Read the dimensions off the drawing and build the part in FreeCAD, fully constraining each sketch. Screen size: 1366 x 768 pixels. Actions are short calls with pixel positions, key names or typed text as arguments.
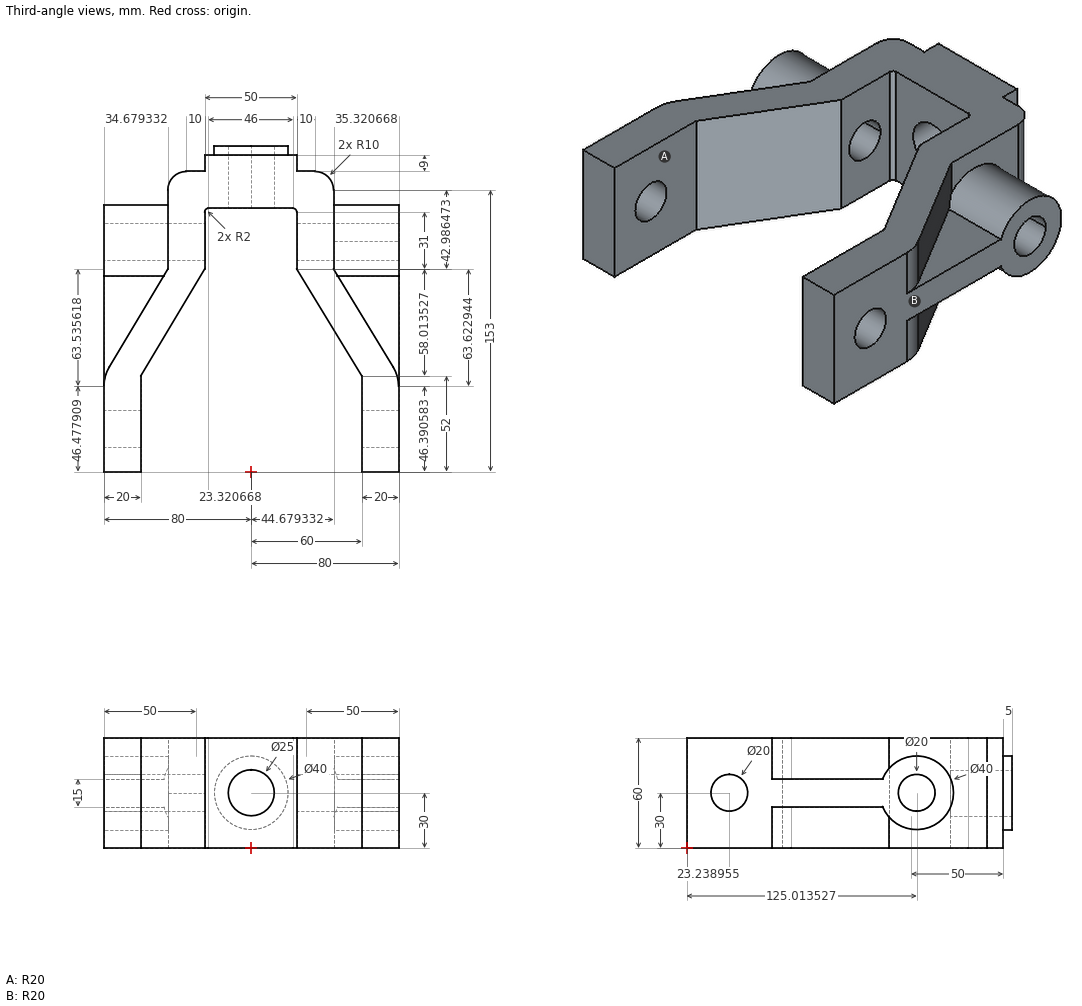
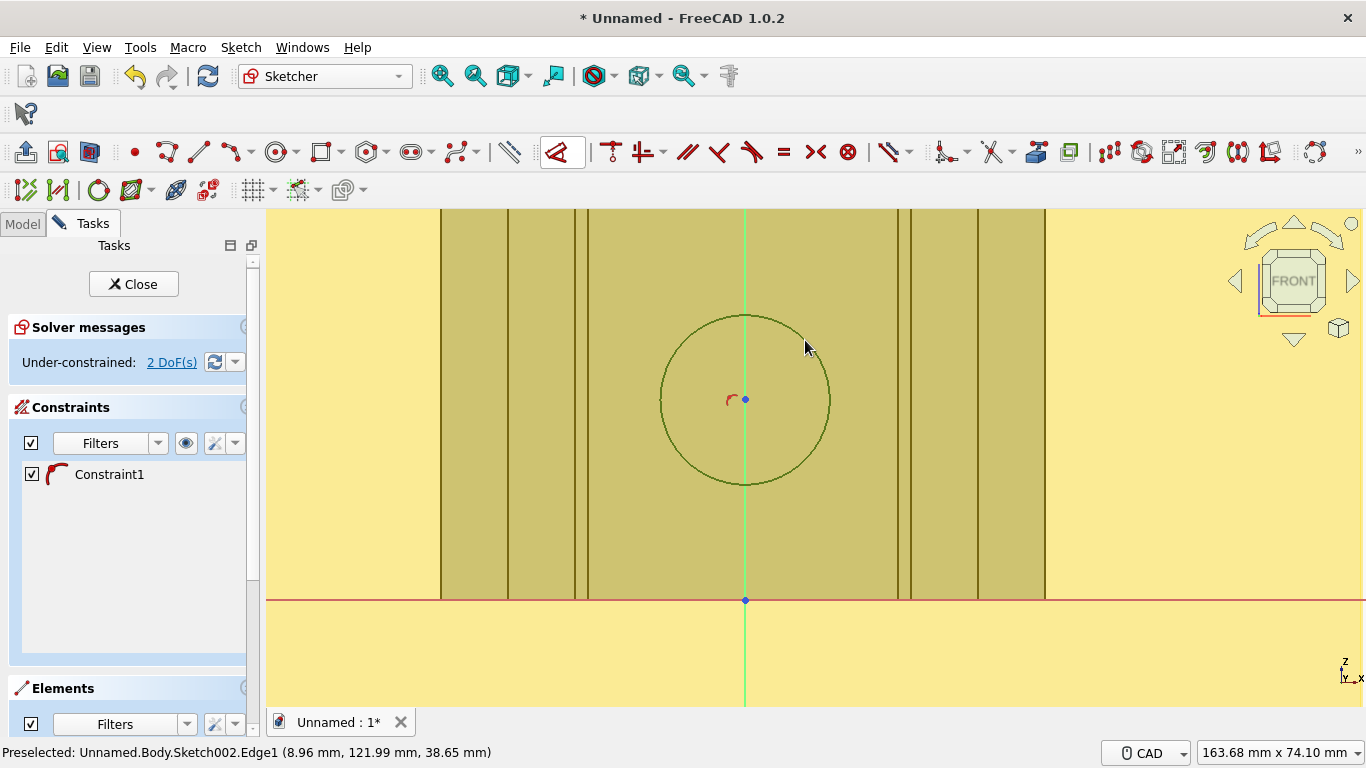
key(k)
key(o)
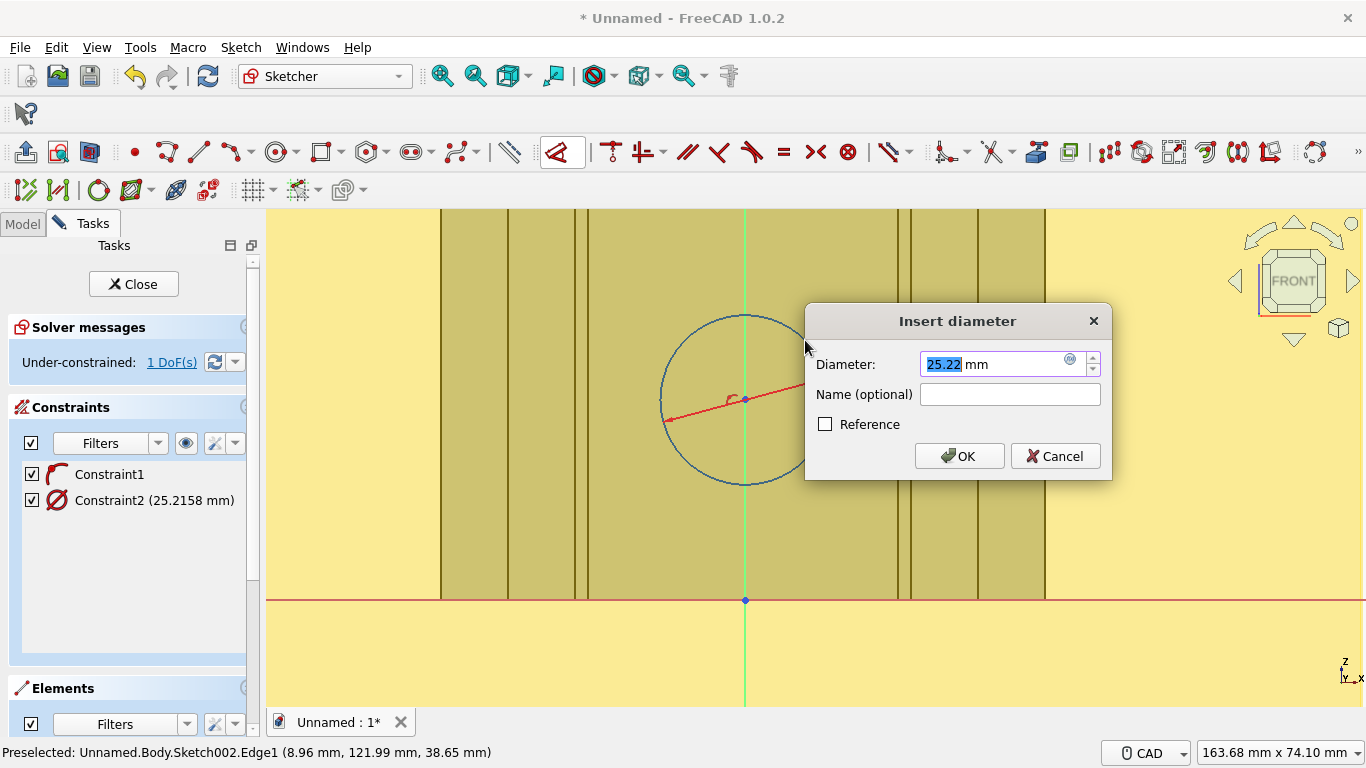
text(25)
key(Return)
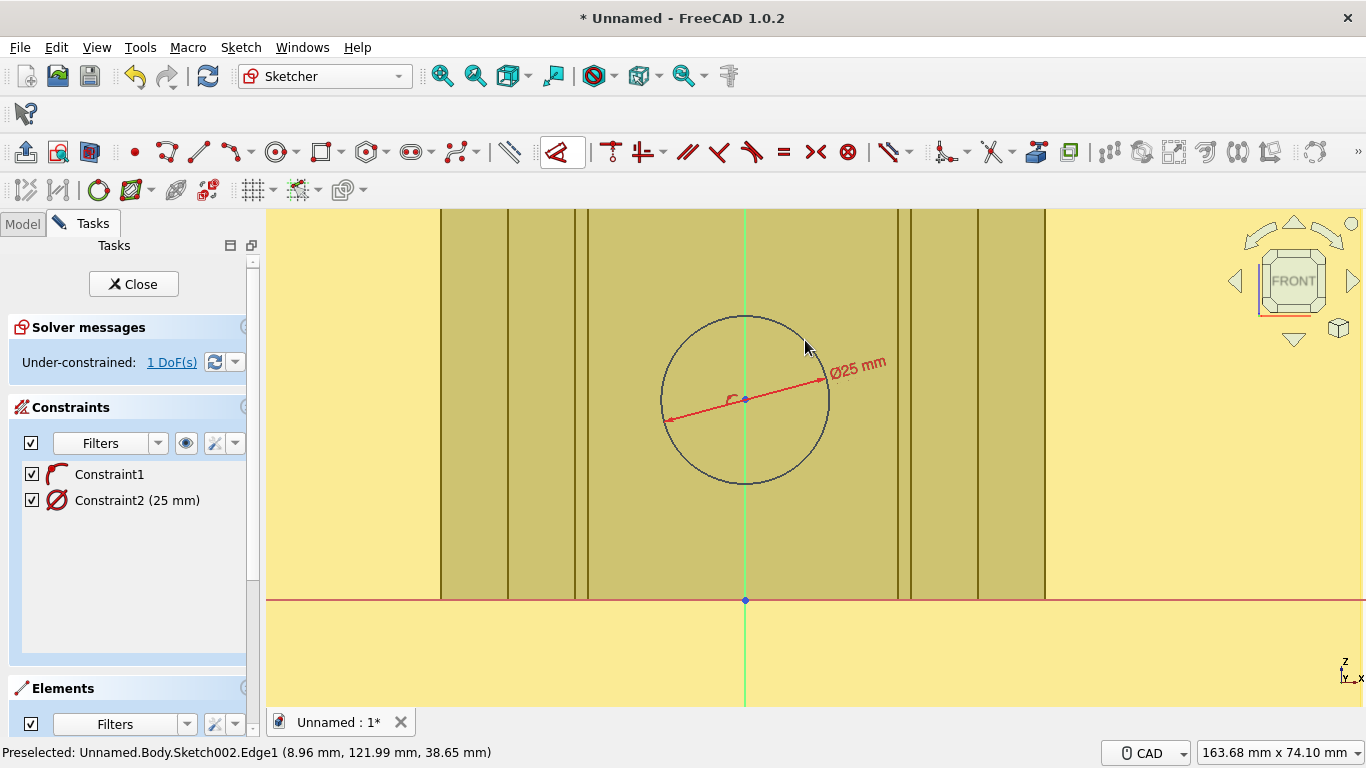
click(745, 400)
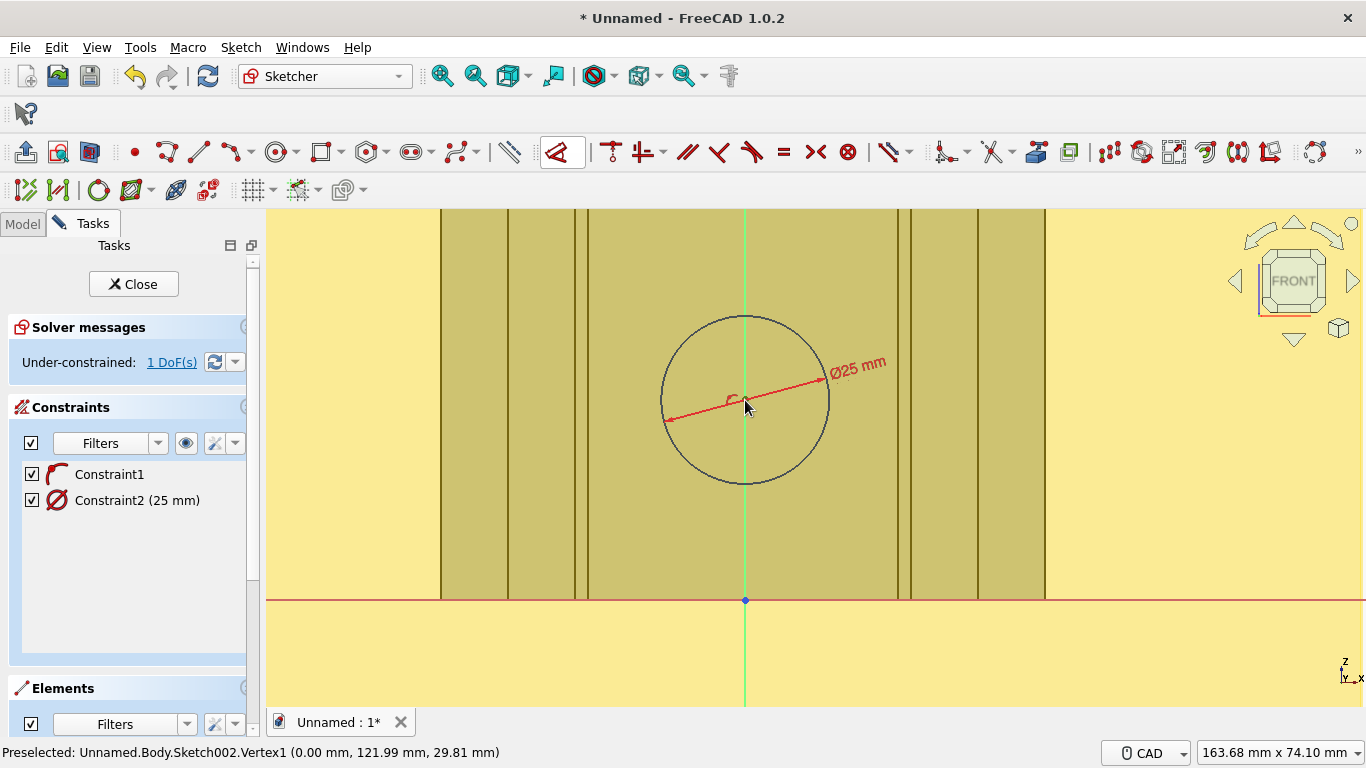
key(i)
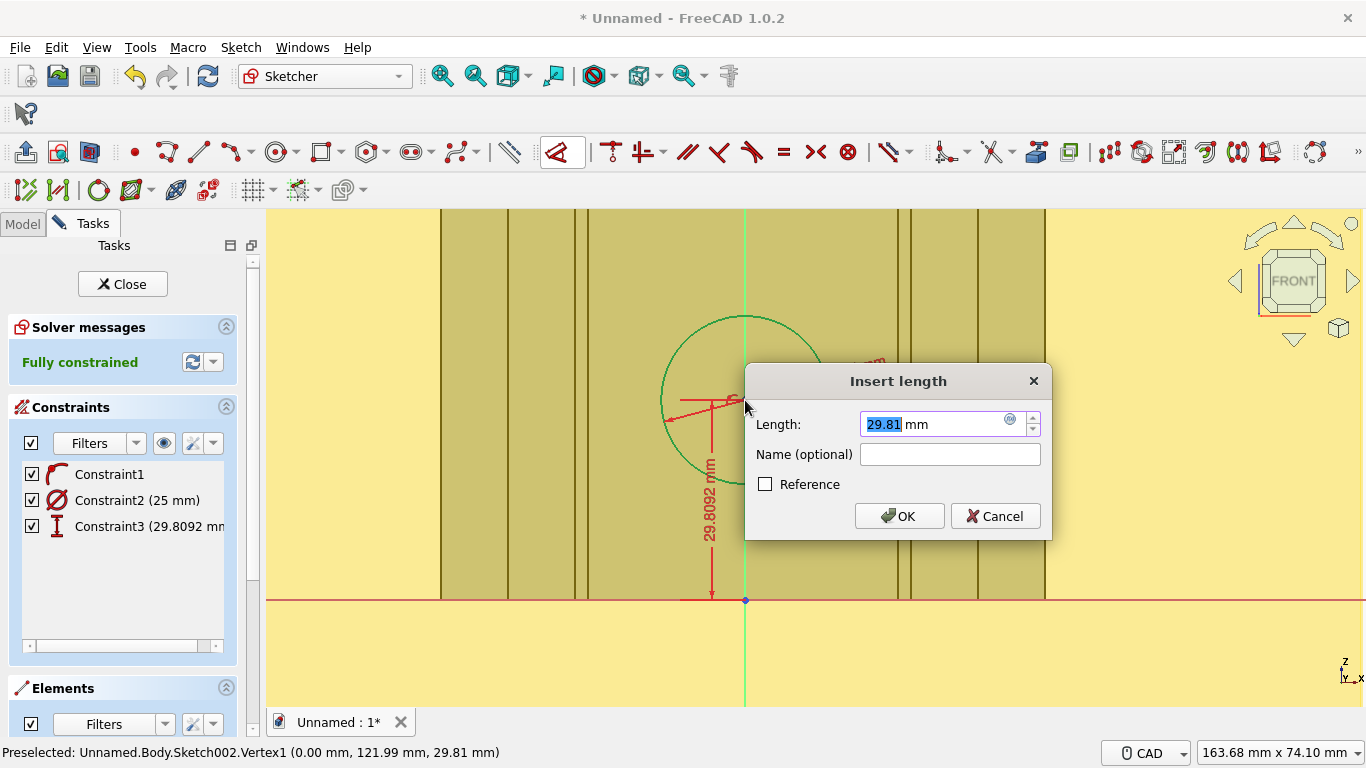
text(30)
key(Return)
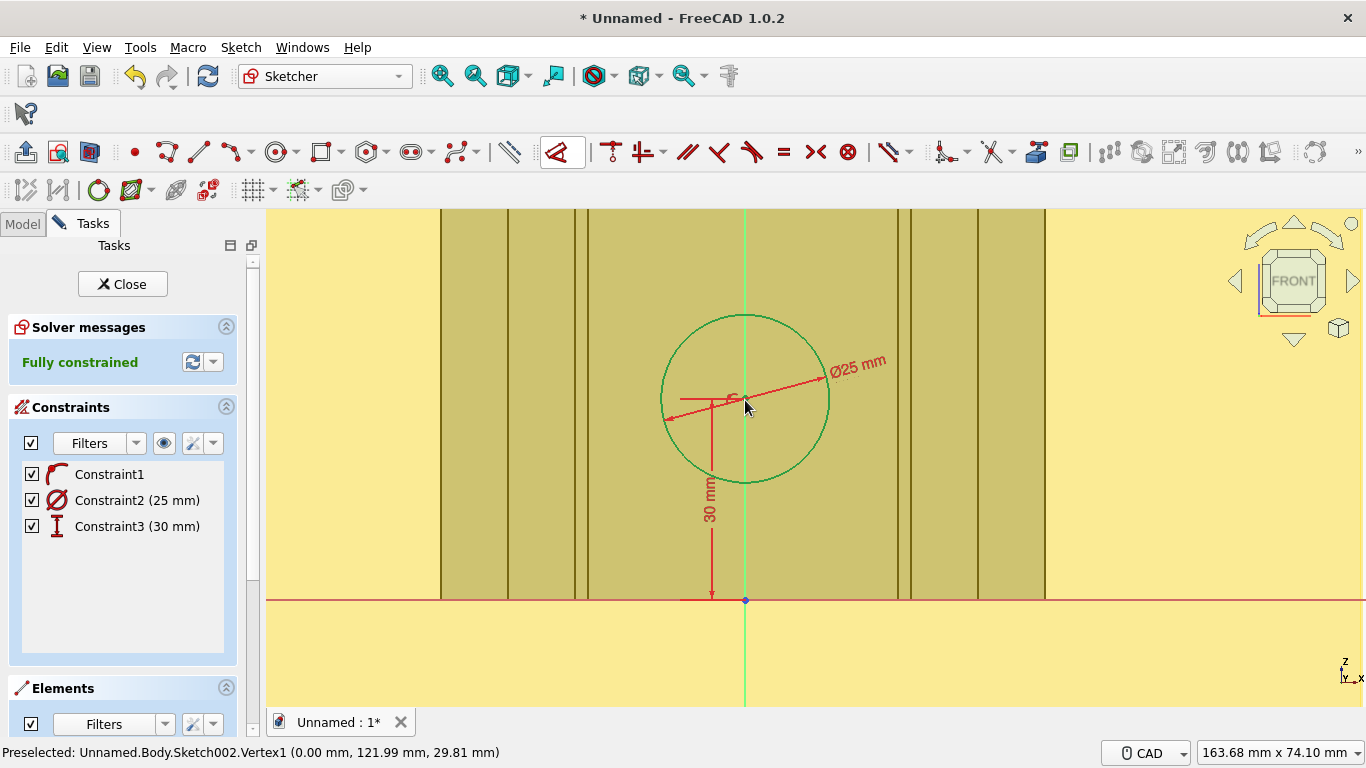
click(123, 284)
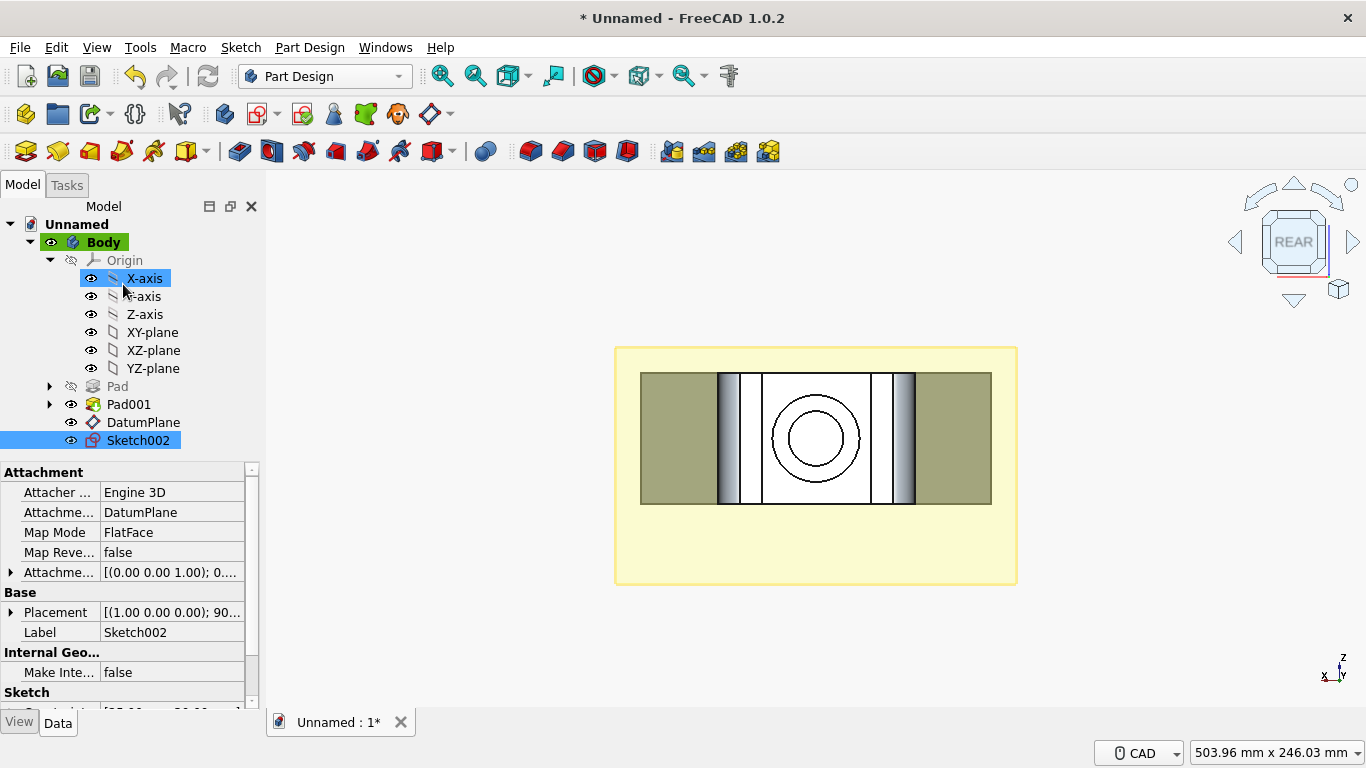
click(240, 152)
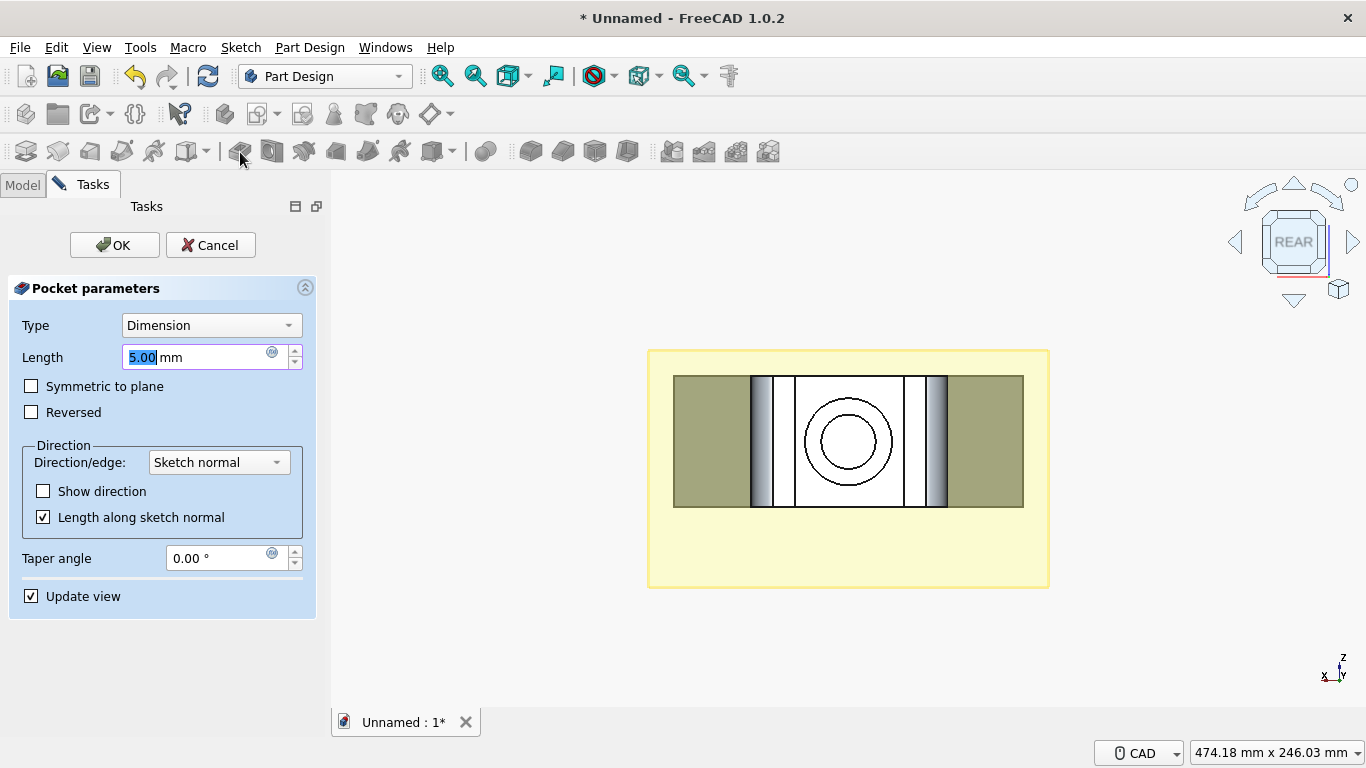
text(50)
key(Tab)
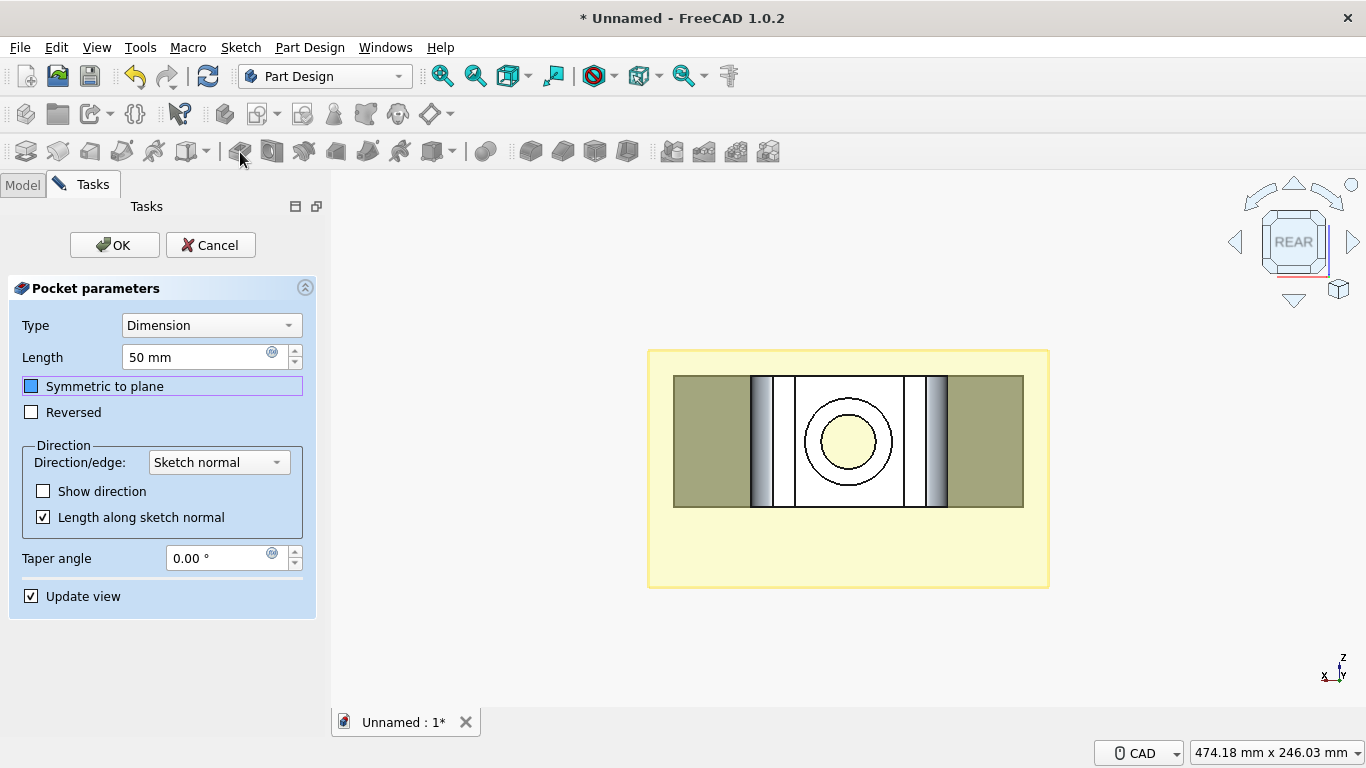
click(115, 245)